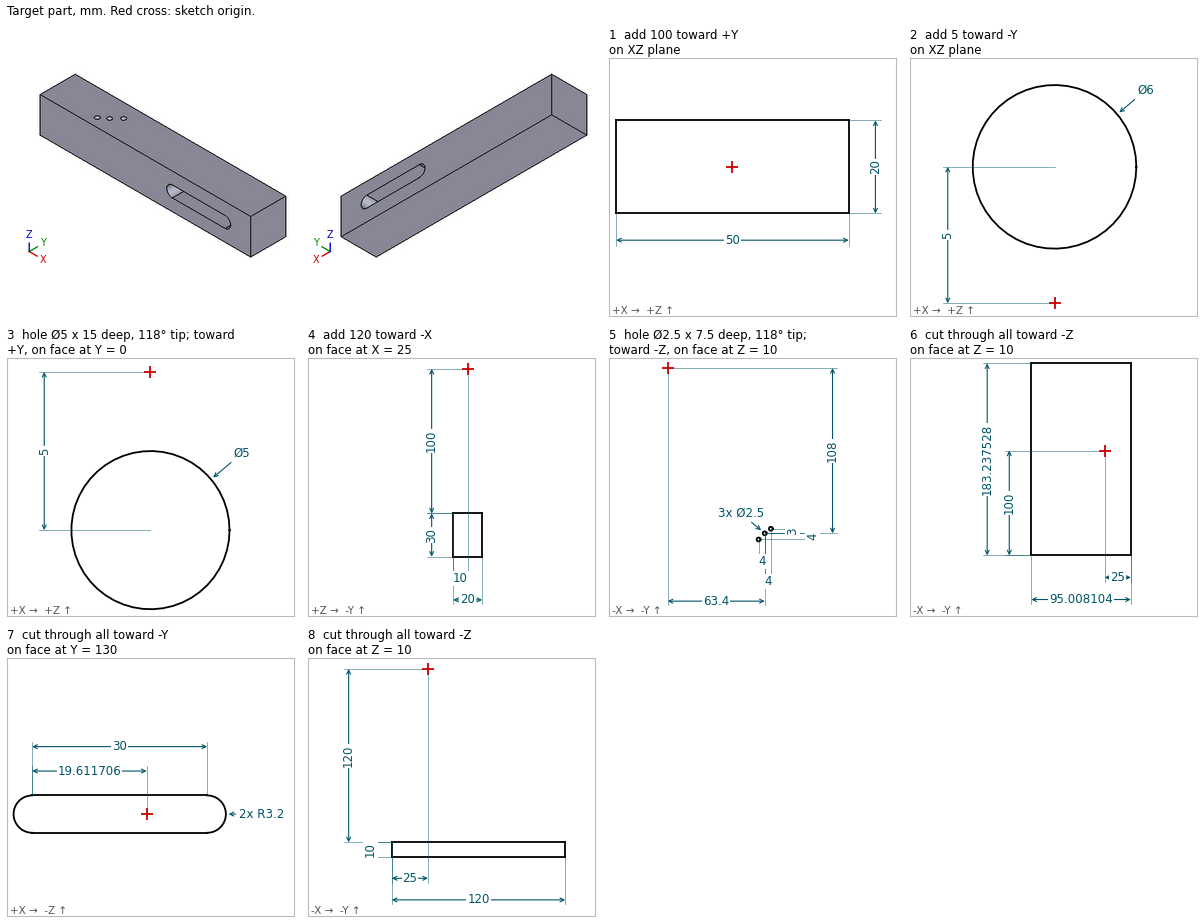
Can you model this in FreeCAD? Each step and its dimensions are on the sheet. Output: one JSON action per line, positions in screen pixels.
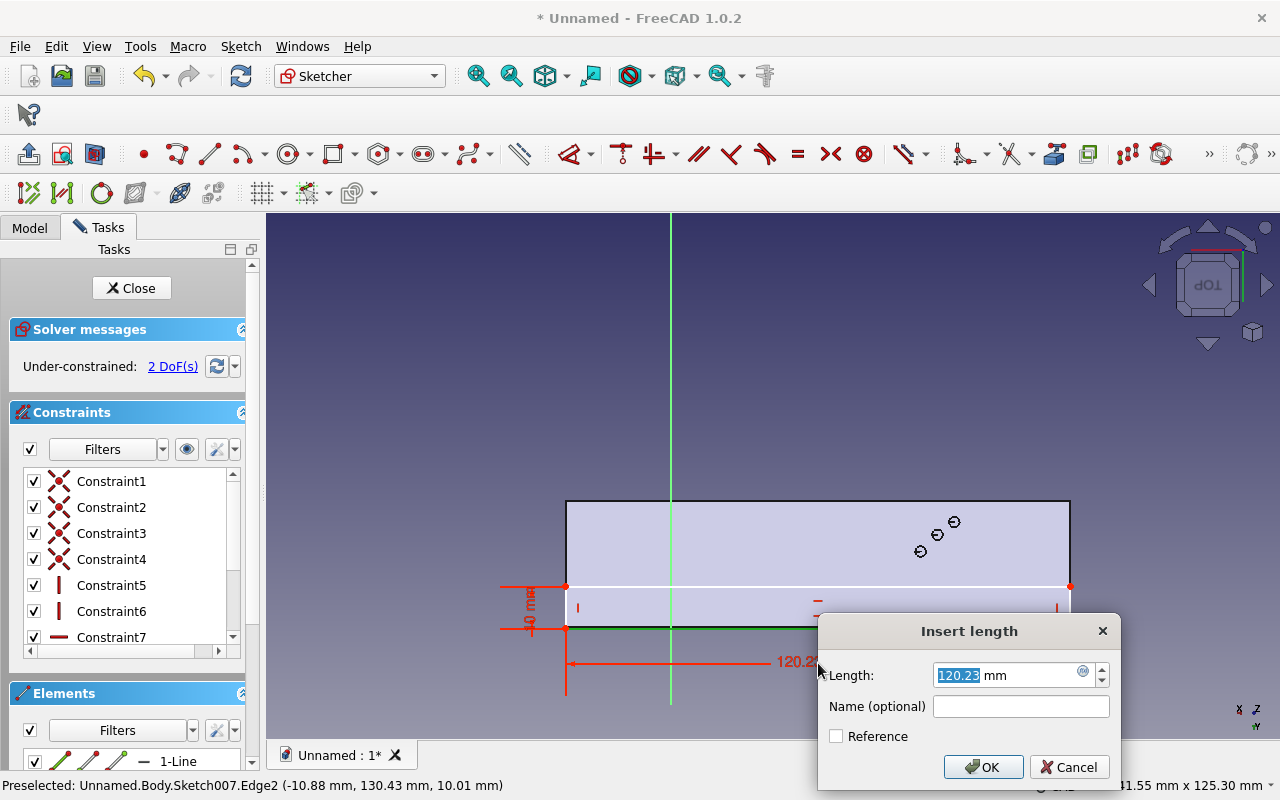
{"action": "type", "text": "120"}
{"action": "key", "text": "Return"}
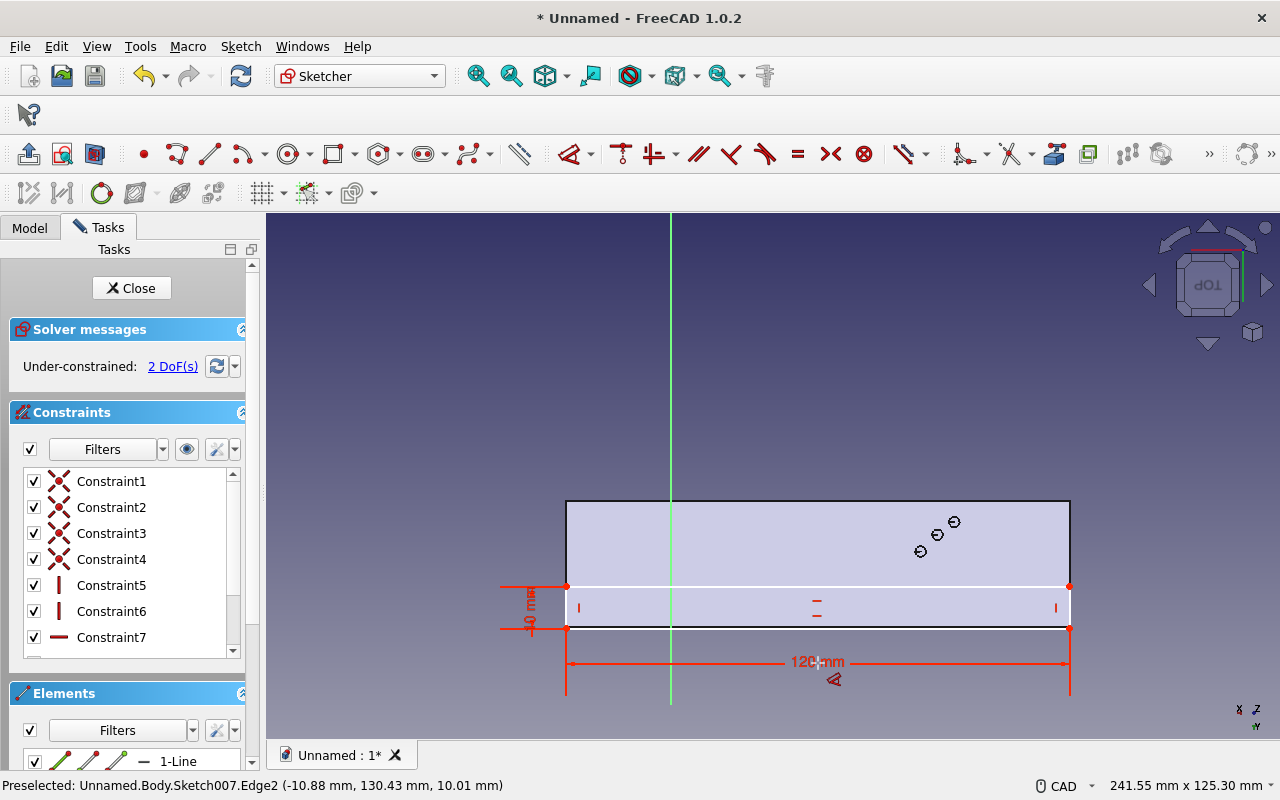
{"action": "left_click", "coordinate": [566, 587]}
{"action": "left_click", "coordinate": [619, 645]}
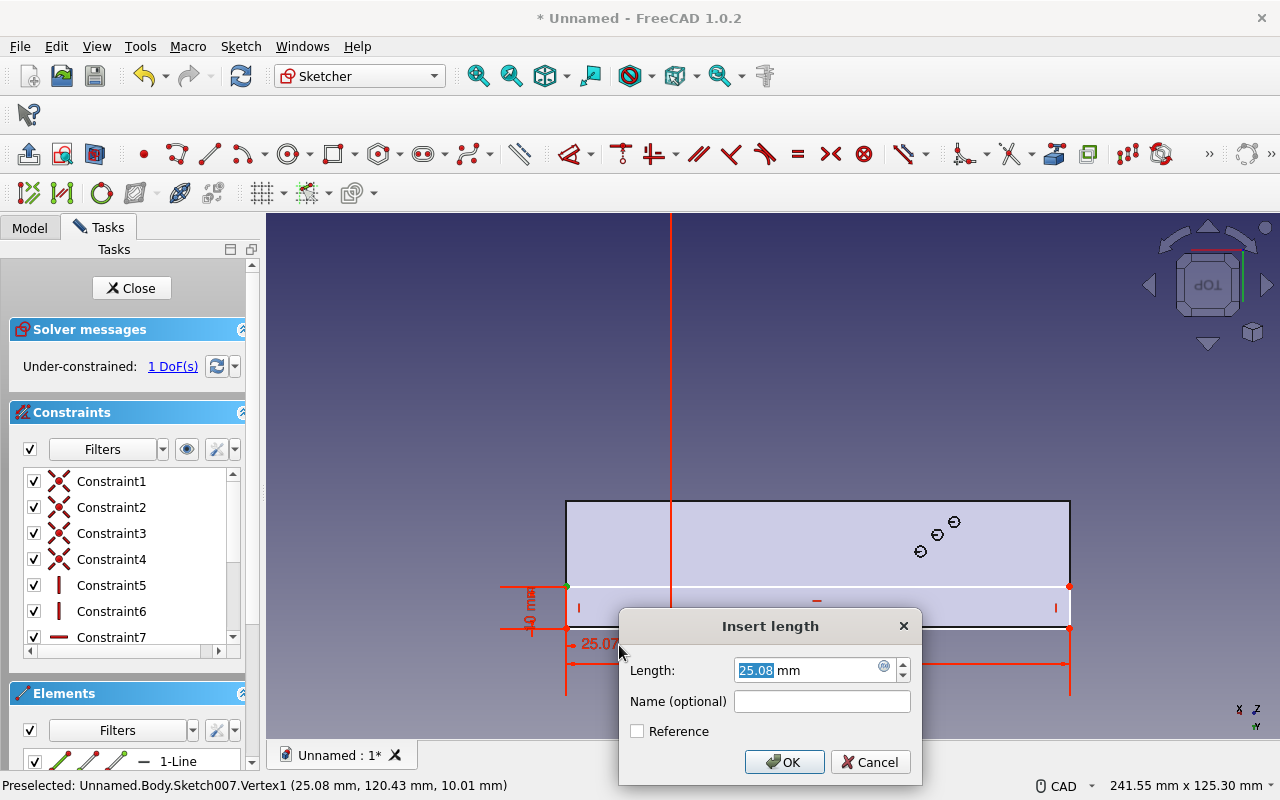
{"action": "type", "text": "25"}
{"action": "key", "text": "Return"}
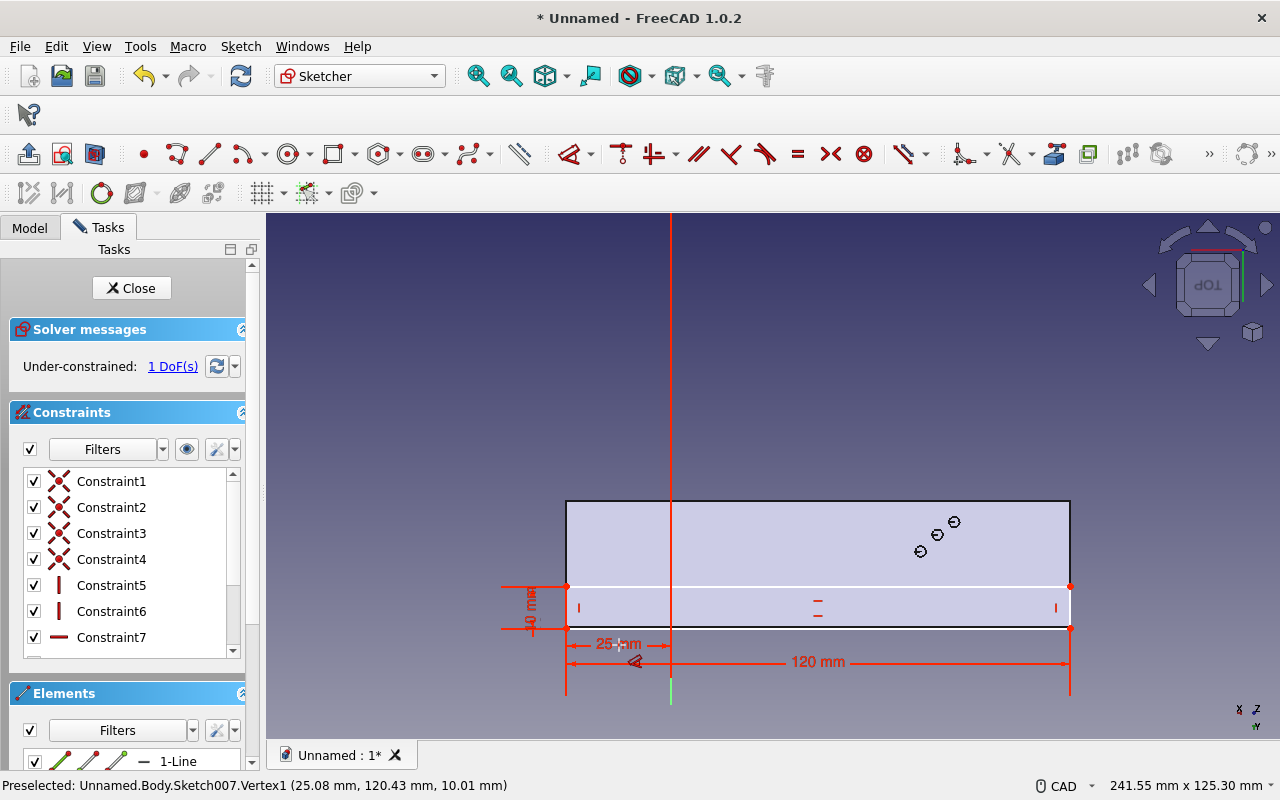
{"action": "left_click", "coordinate": [566, 587]}
{"action": "left_click", "coordinate": [532, 414]}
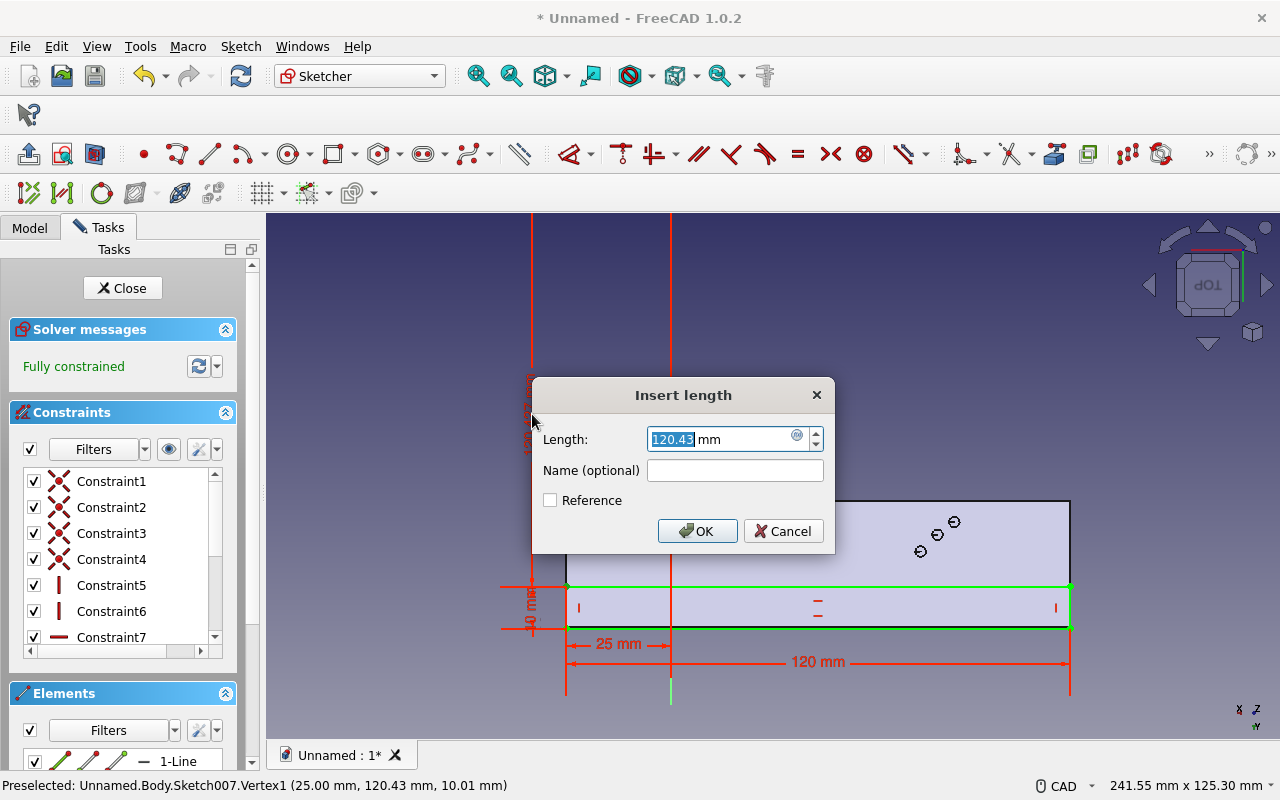
{"action": "type", "text": "120"}
{"action": "key", "text": "Return"}
{"action": "key", "text": "Escape"}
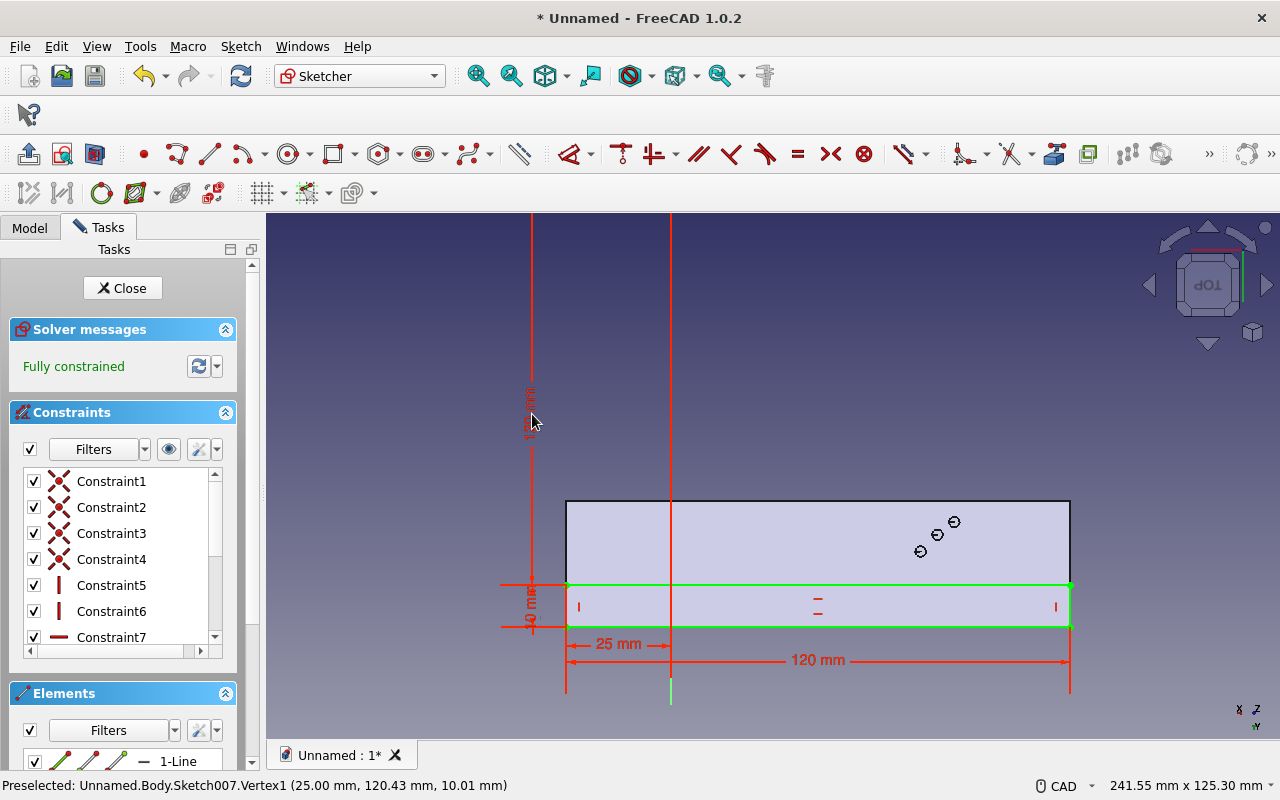
{"action": "left_click", "coordinate": [123, 288]}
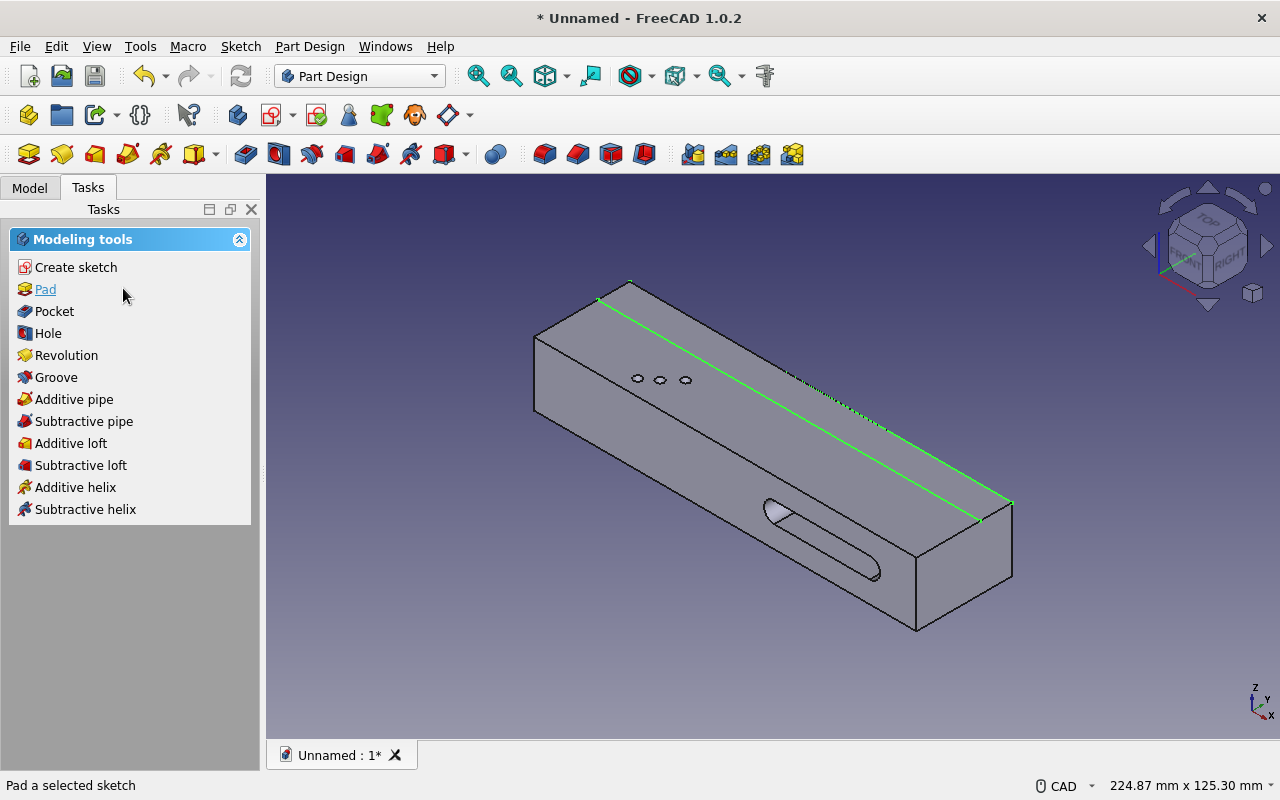
{"action": "left_click", "coordinate": [246, 154]}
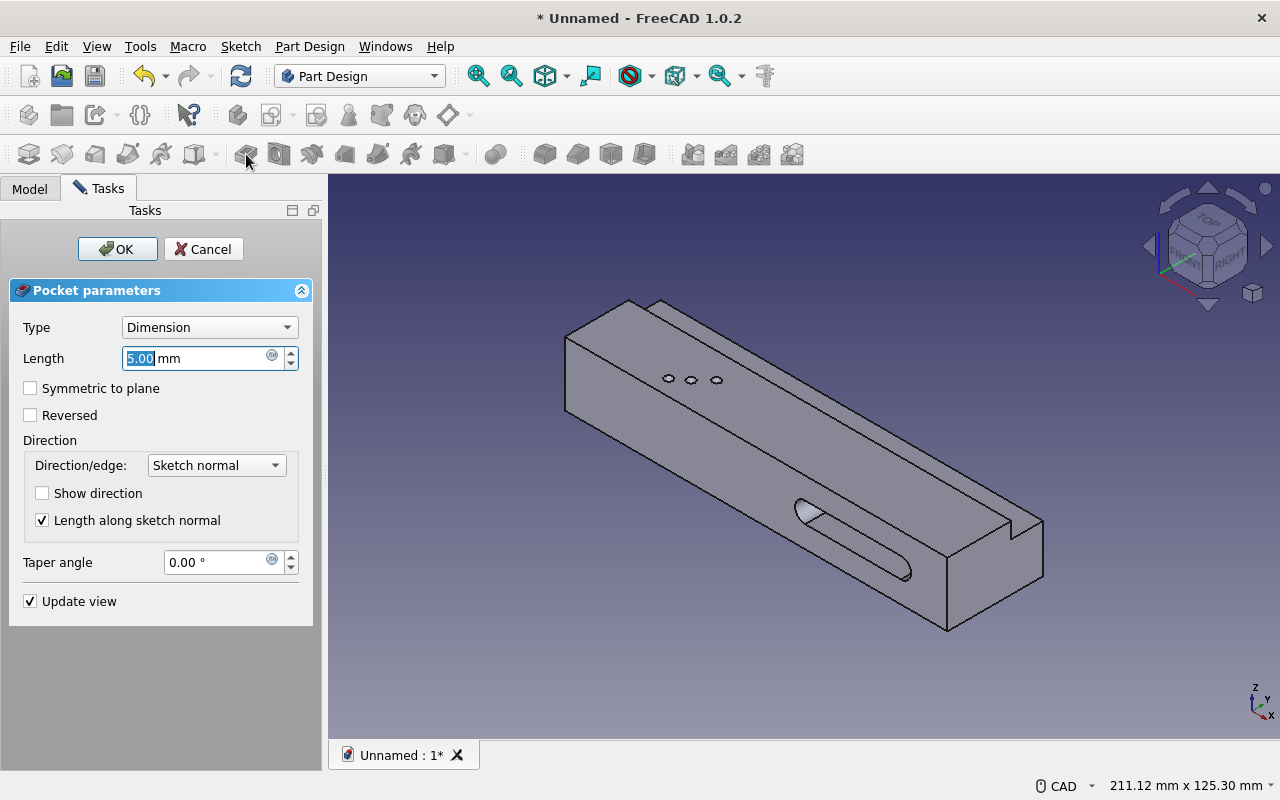
{"action": "left_click", "coordinate": [210, 328]}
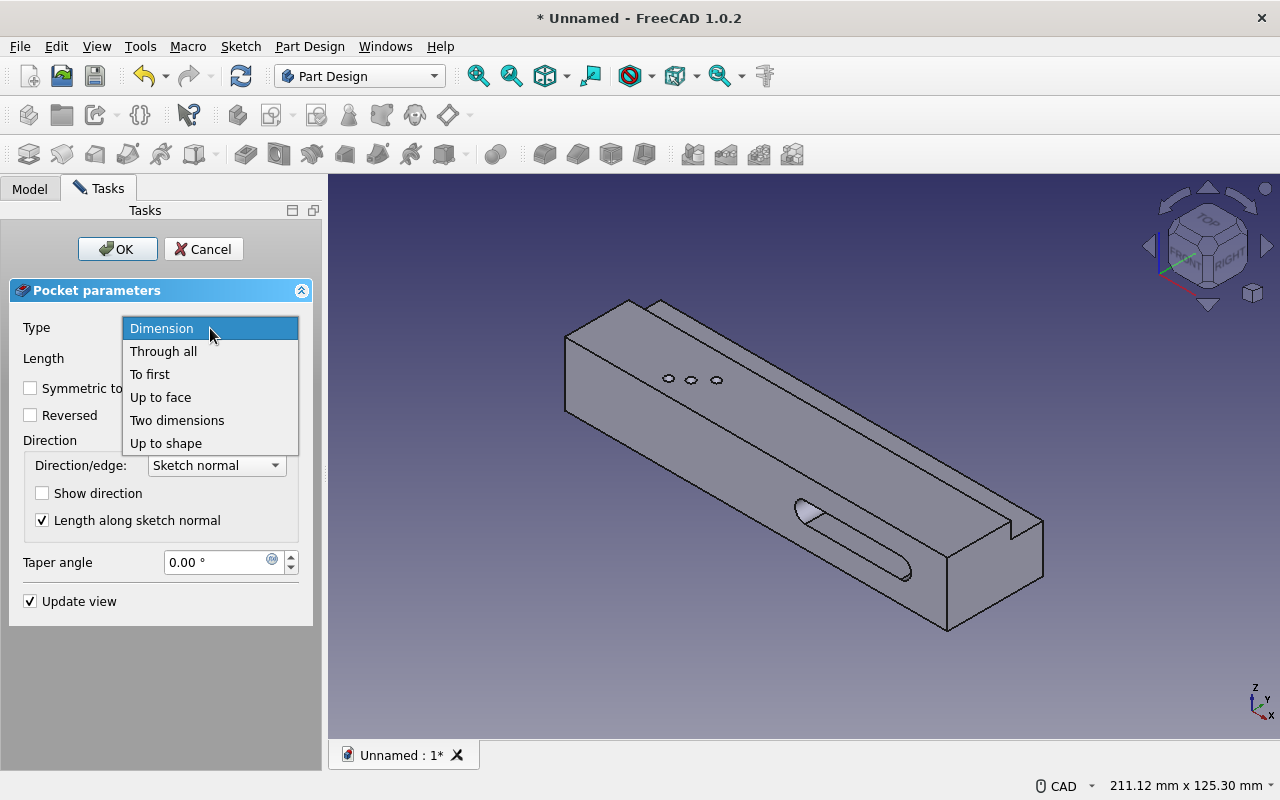
{"action": "left_click", "coordinate": [208, 352]}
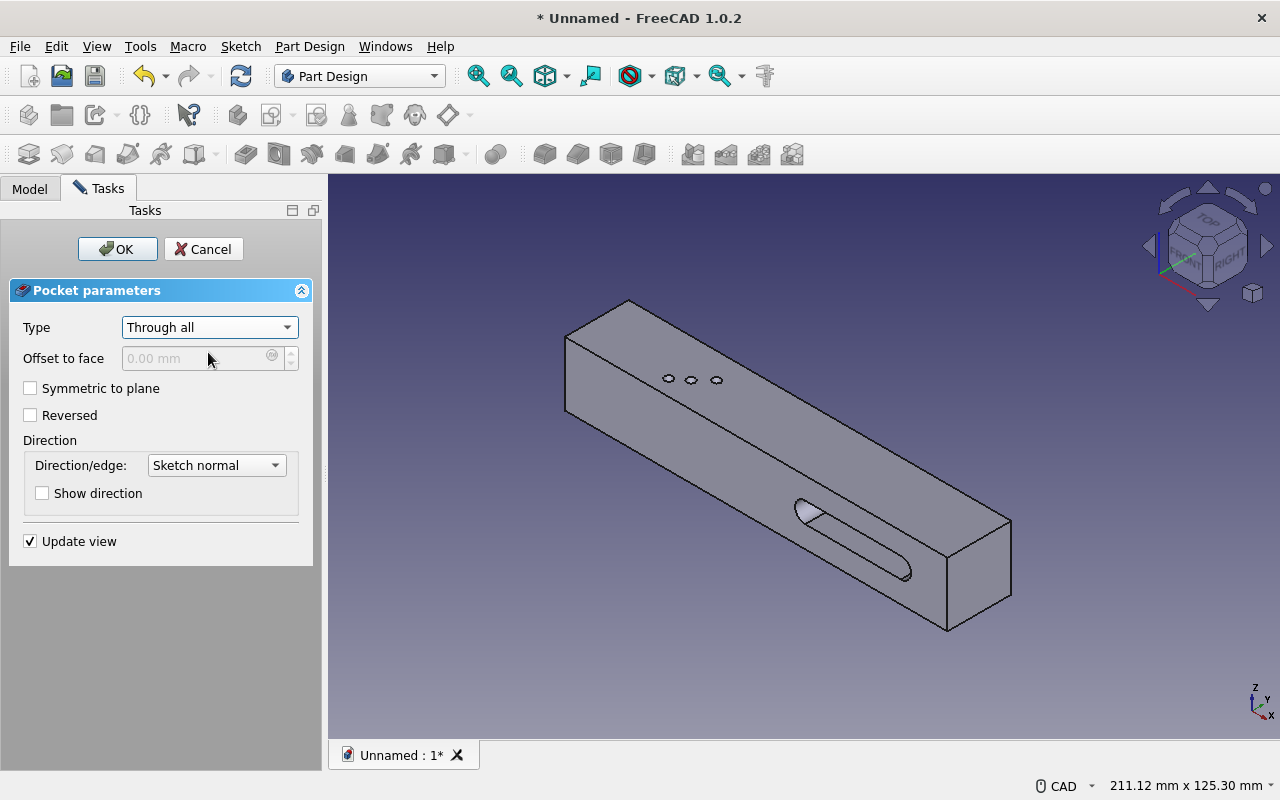
{"action": "left_click", "coordinate": [118, 249]}